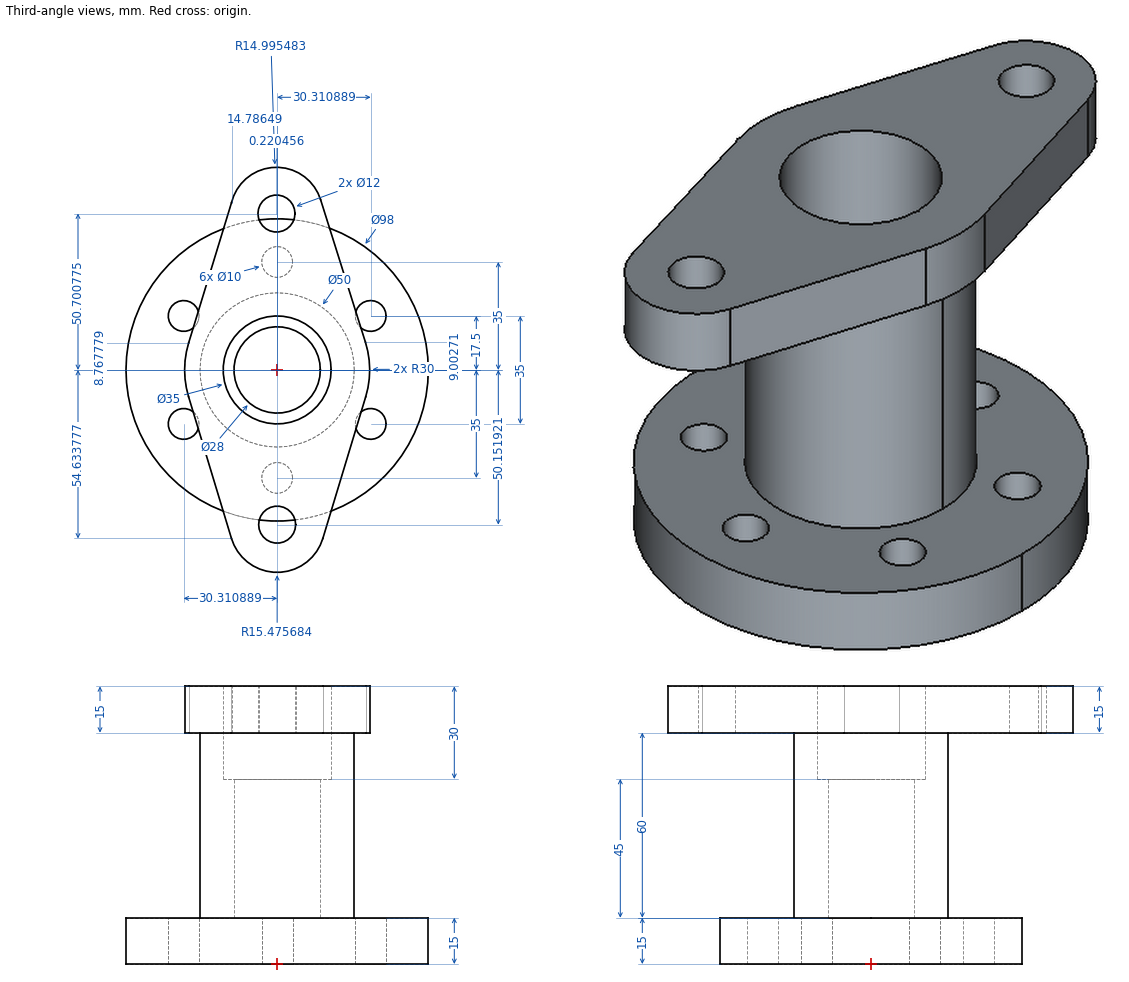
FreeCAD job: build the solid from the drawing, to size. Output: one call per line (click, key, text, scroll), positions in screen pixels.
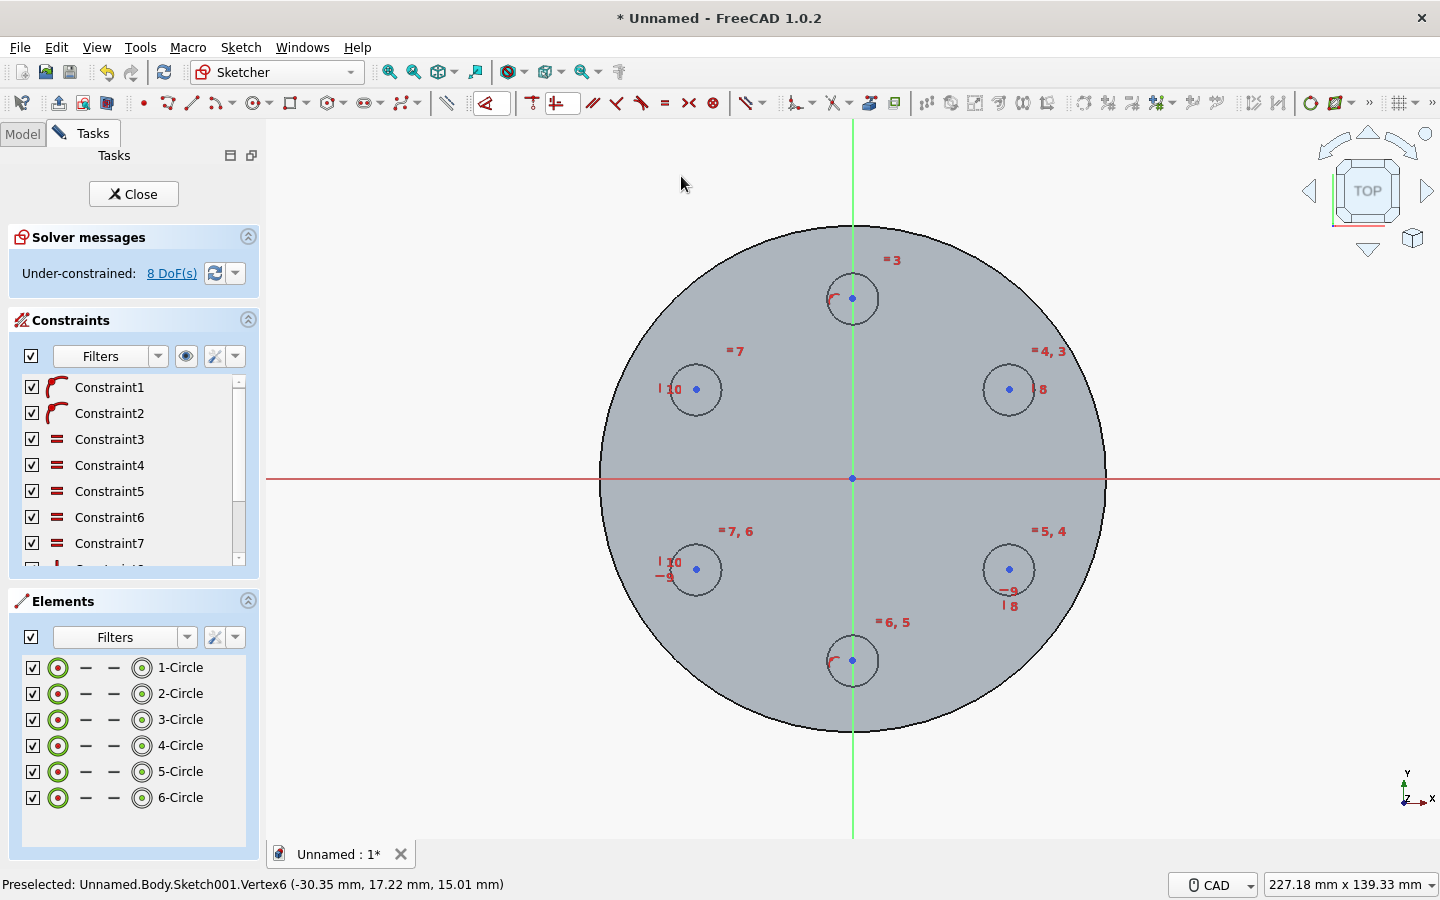
click(1009, 390)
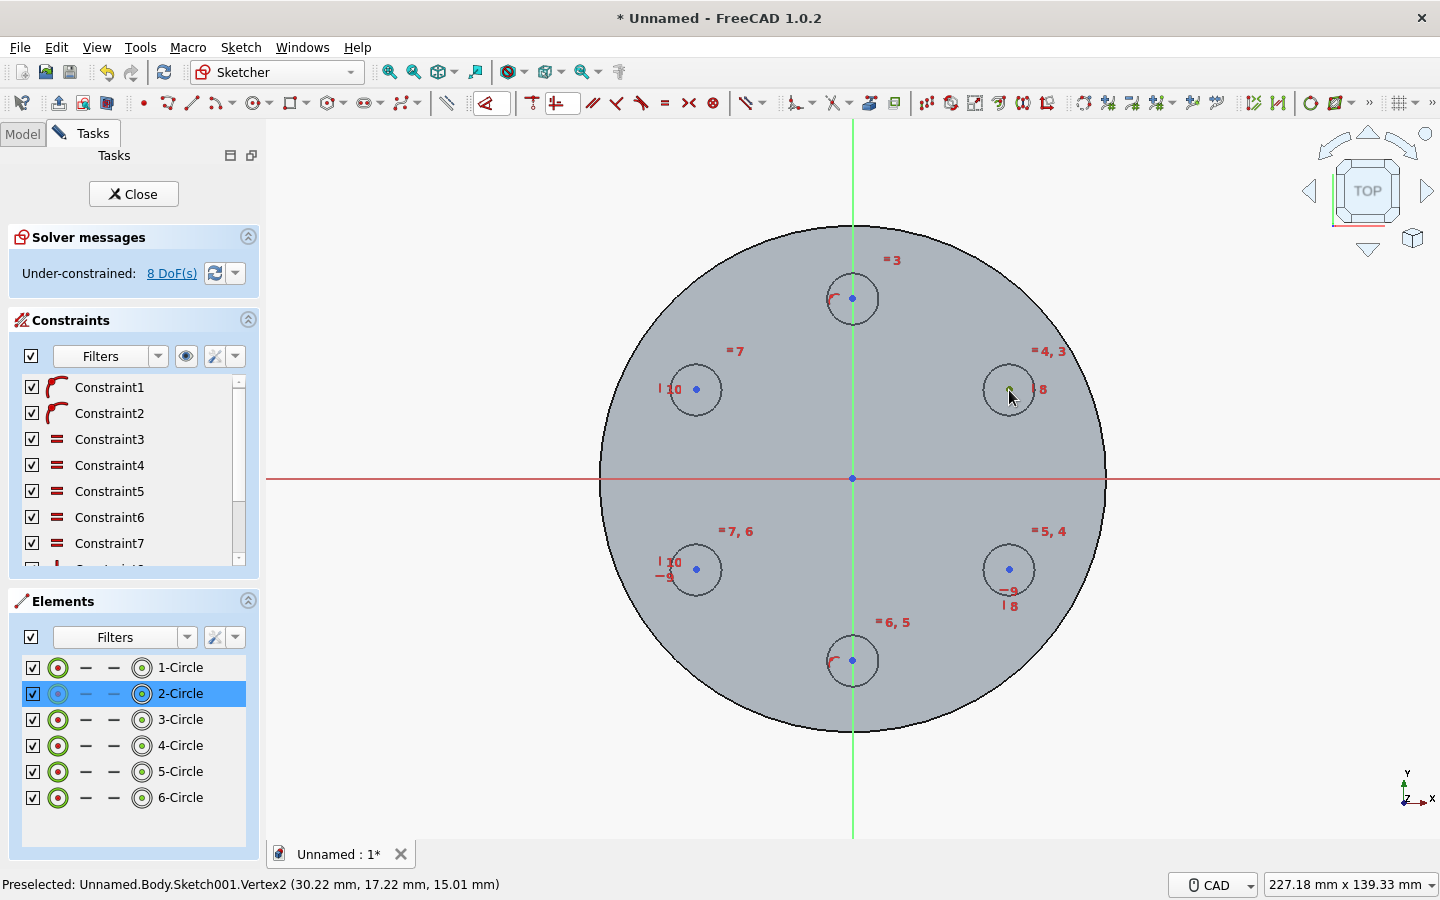
click(696, 390)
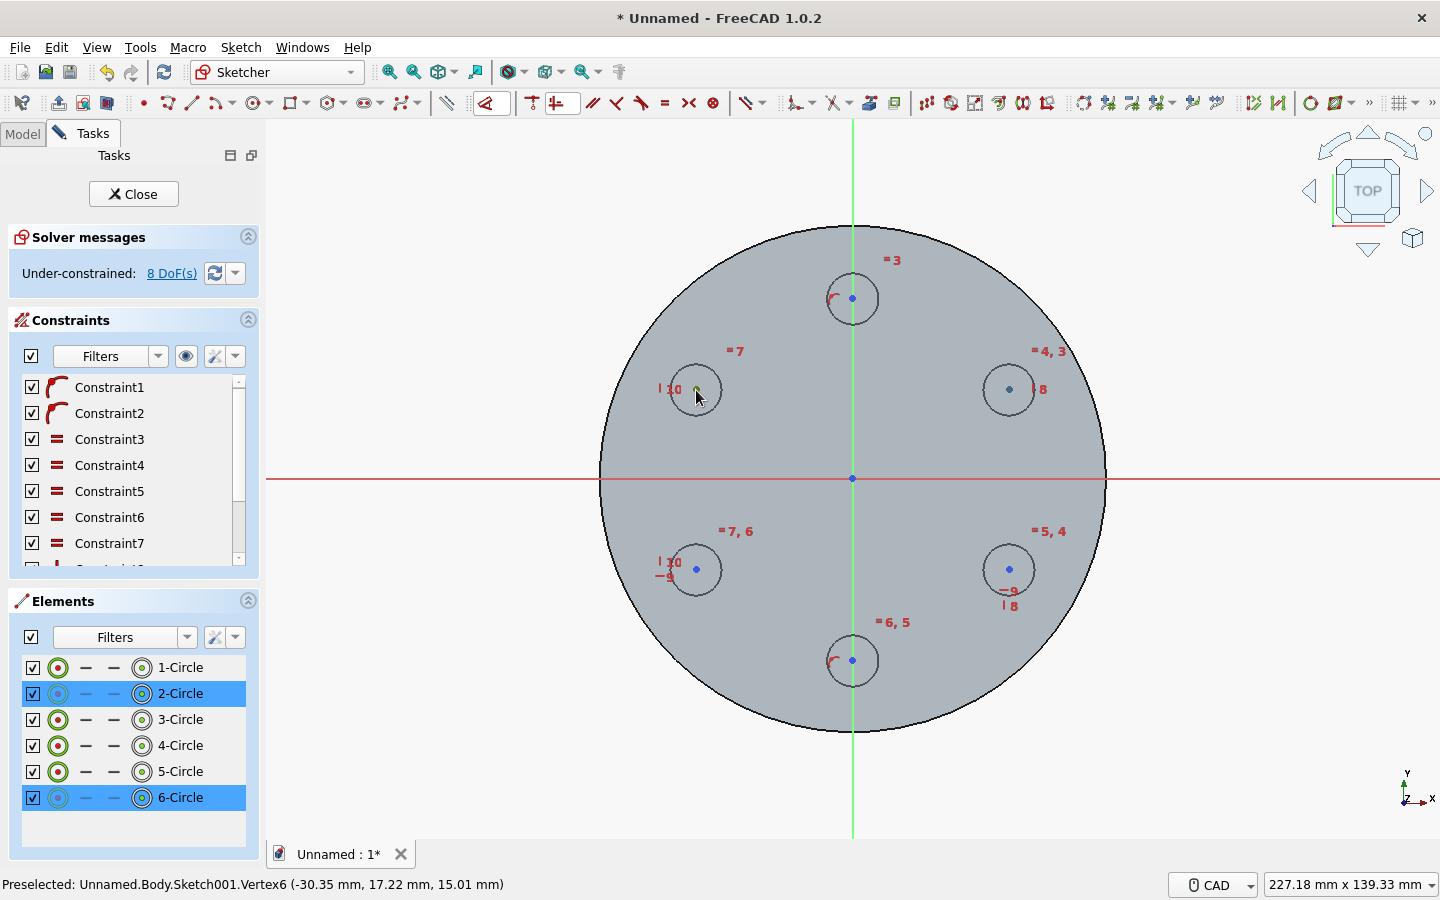
key(h)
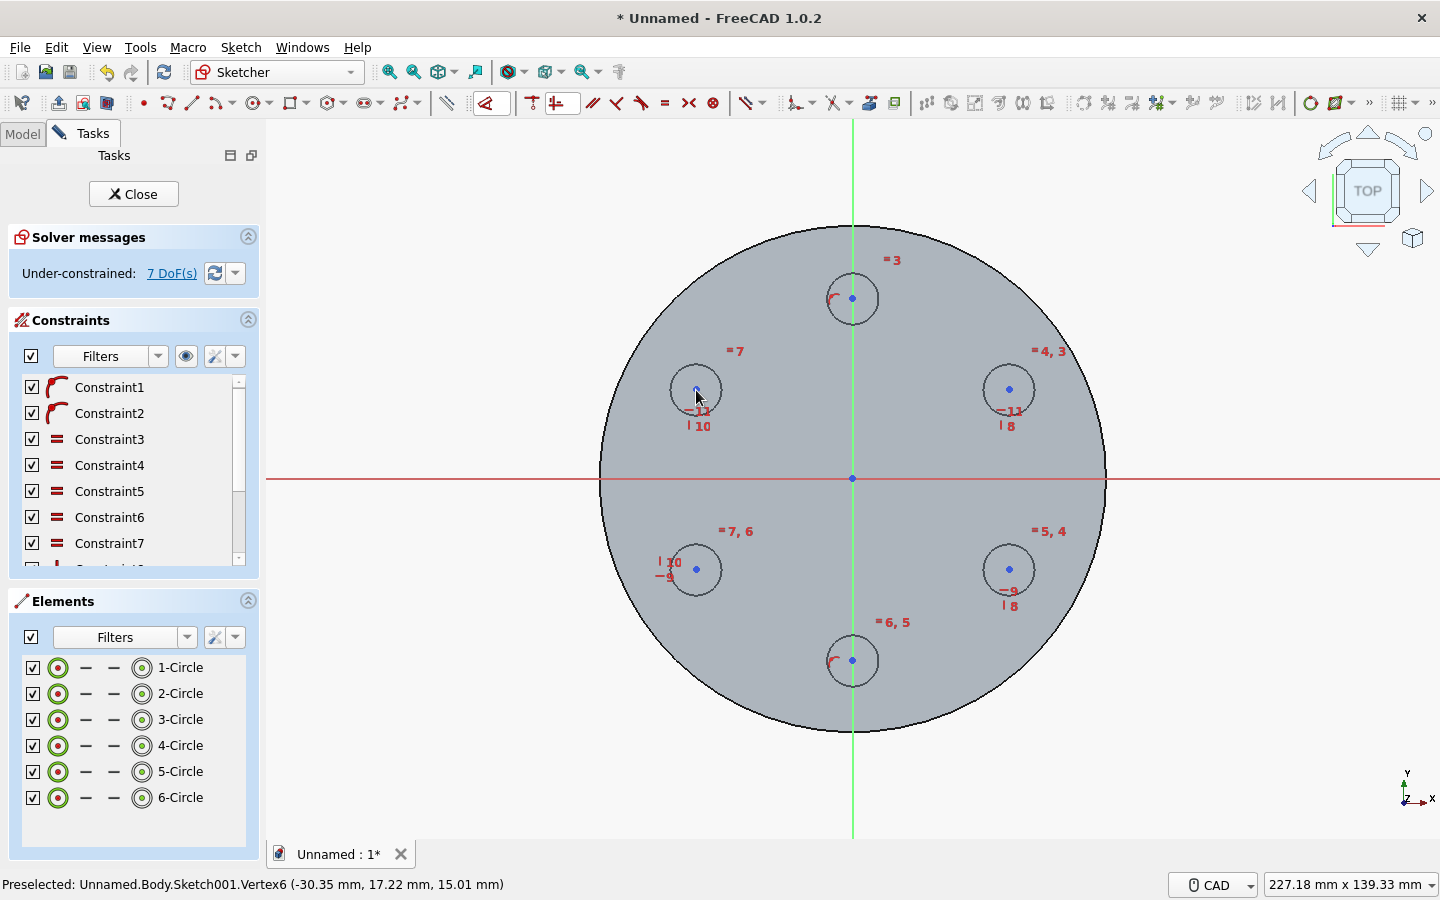
click(871, 281)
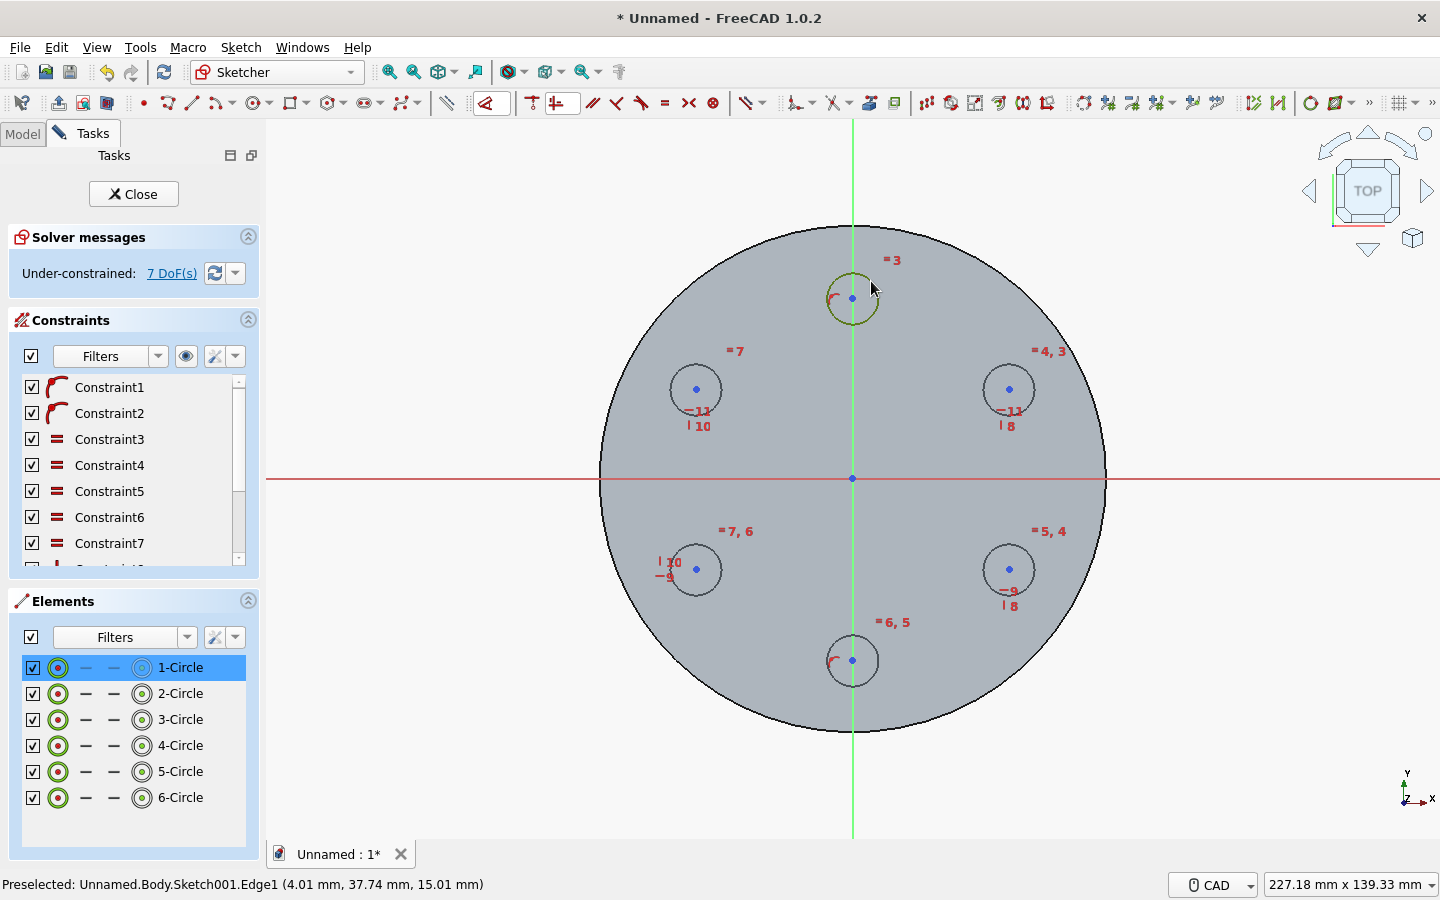
key(k)
key(o)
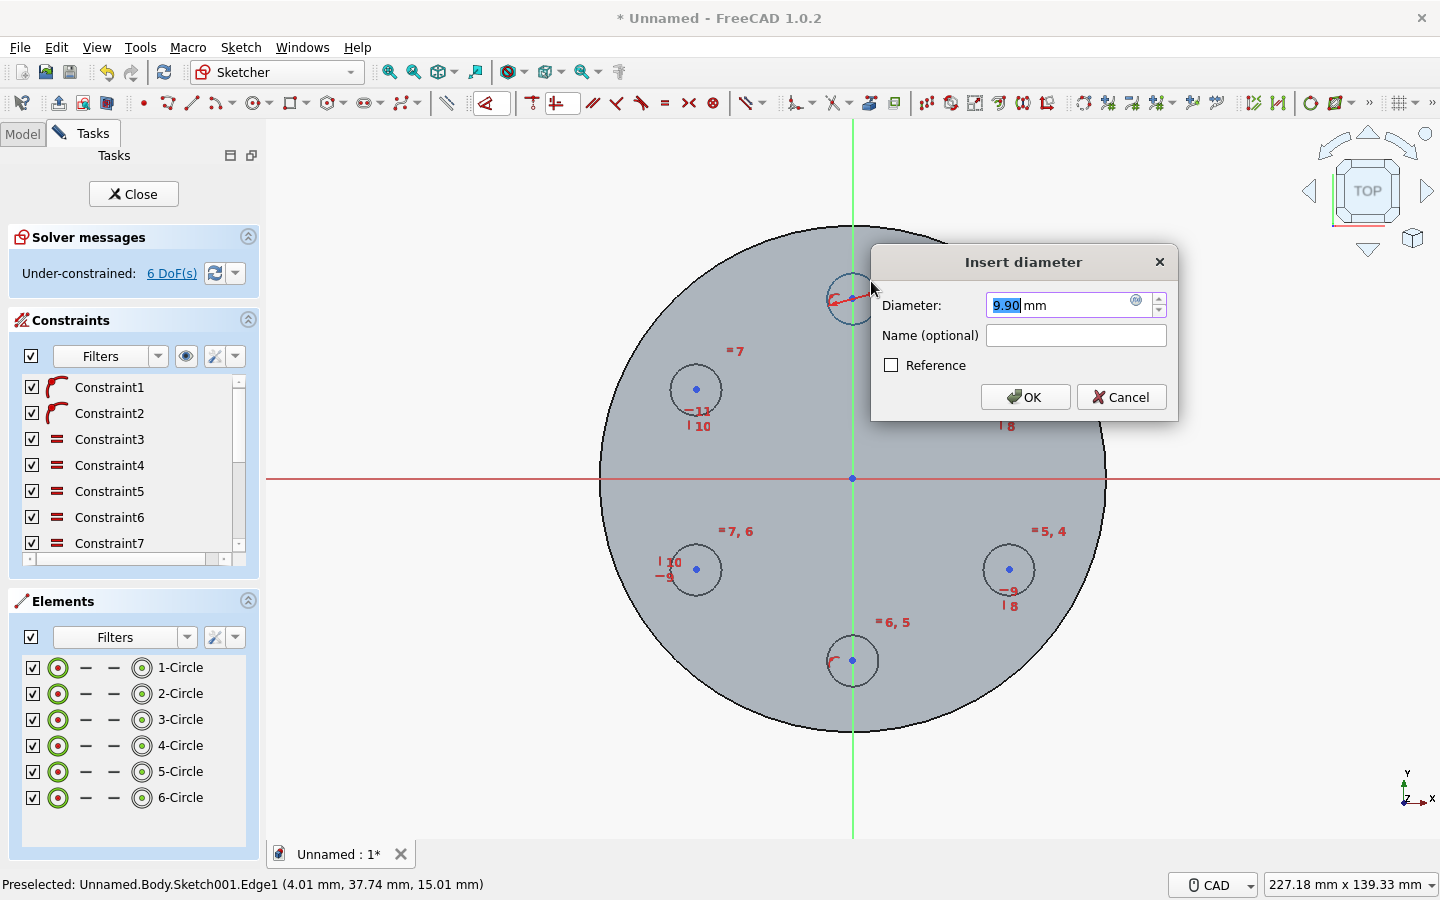
text(10)
key(Return)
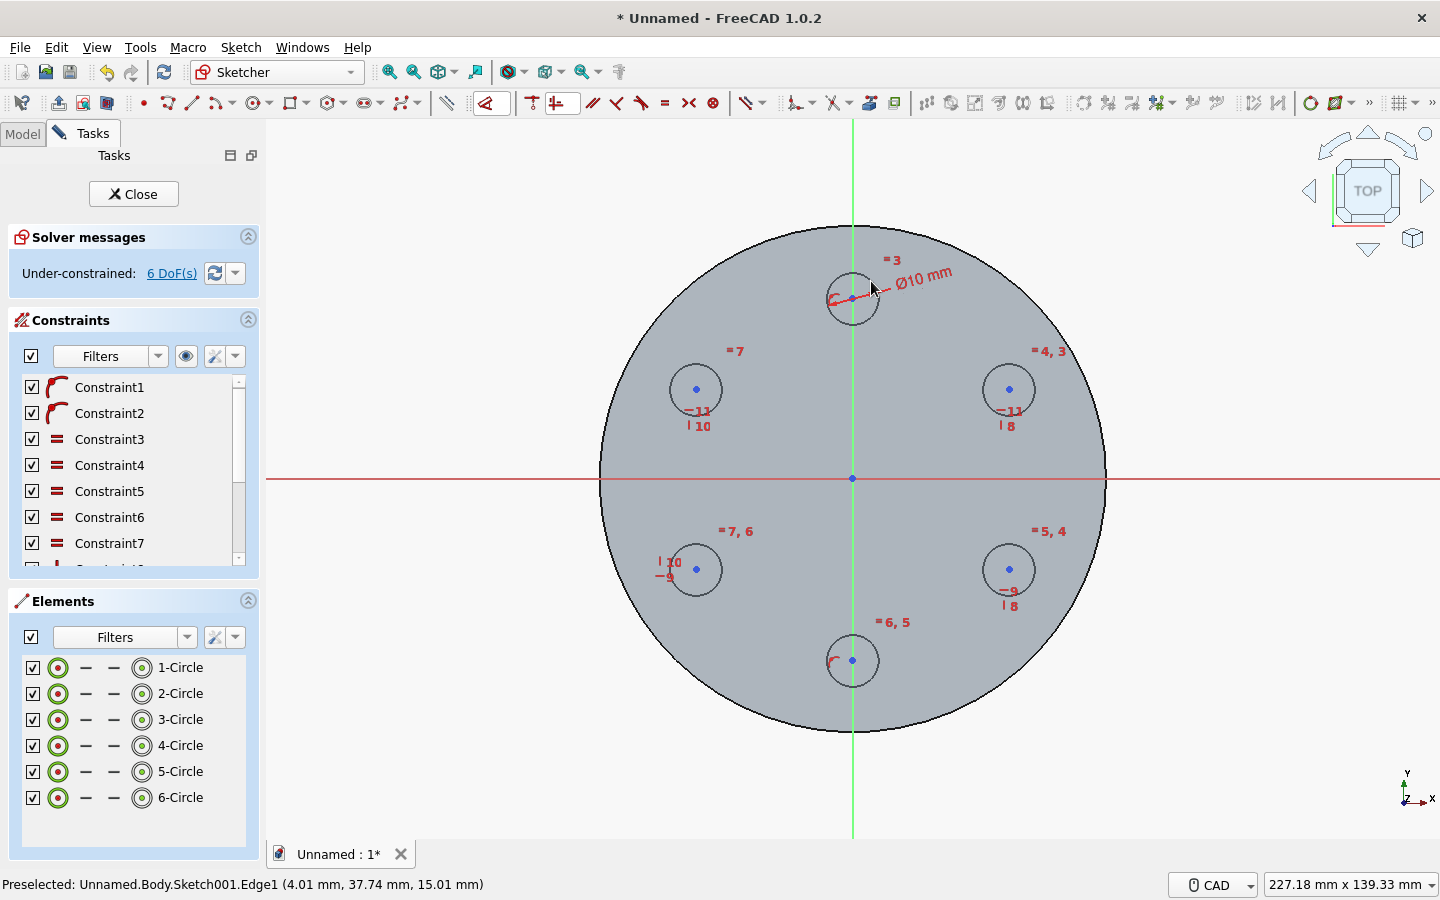
click(853, 299)